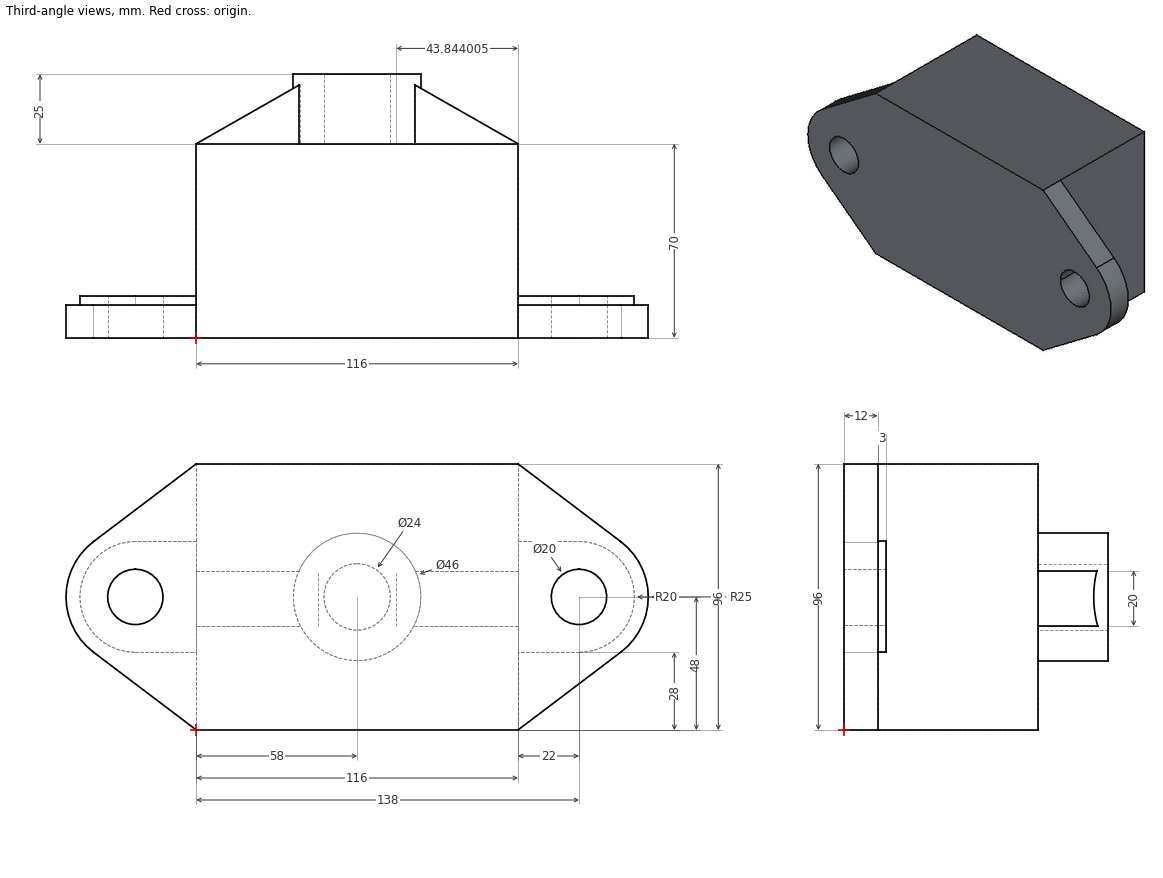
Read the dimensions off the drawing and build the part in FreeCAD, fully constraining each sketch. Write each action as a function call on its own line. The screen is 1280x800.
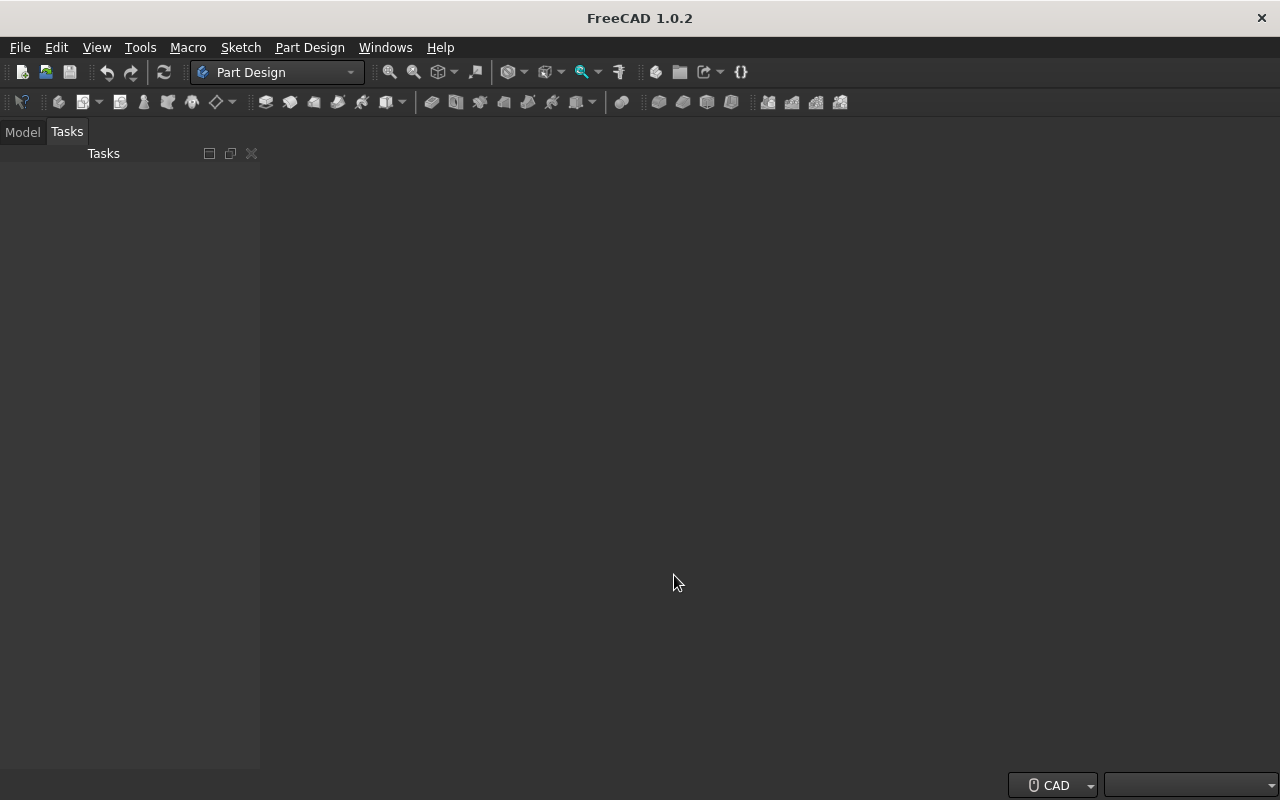
click(22, 72)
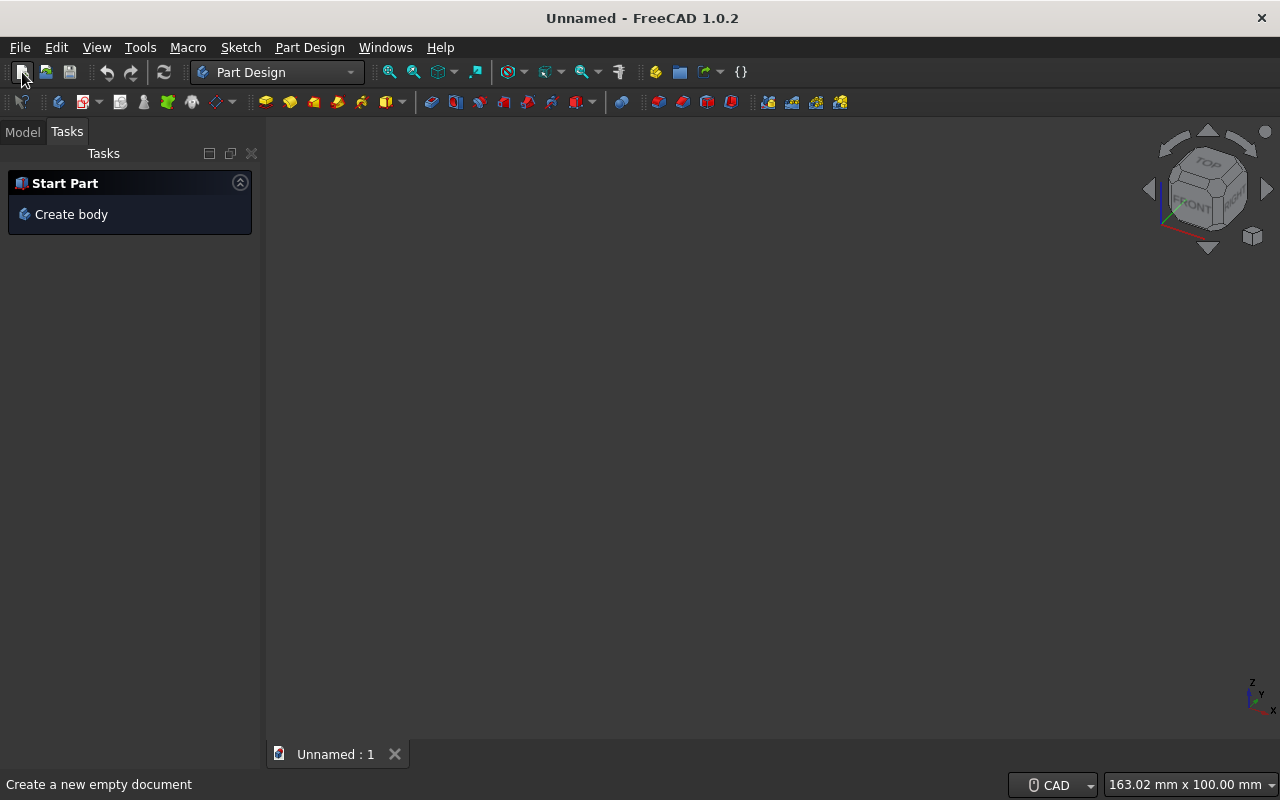
click(84, 102)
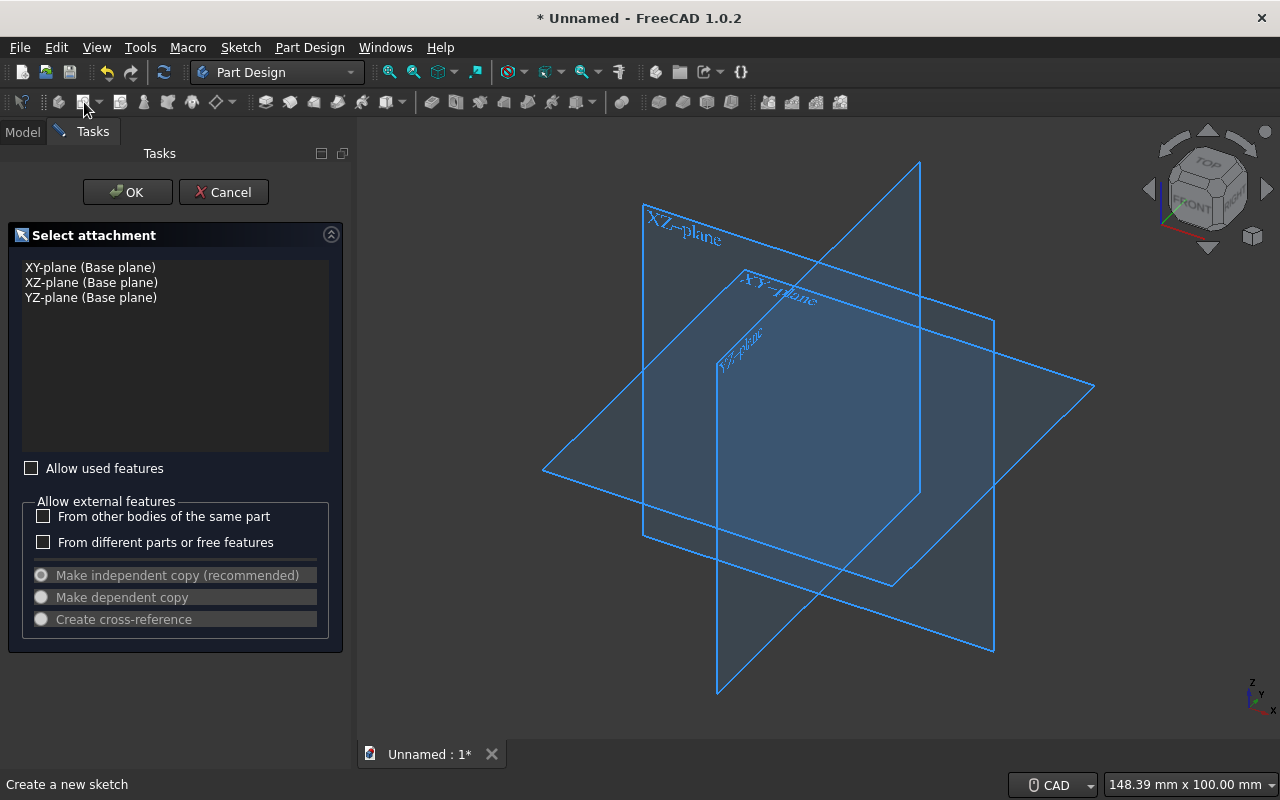
click(82, 268)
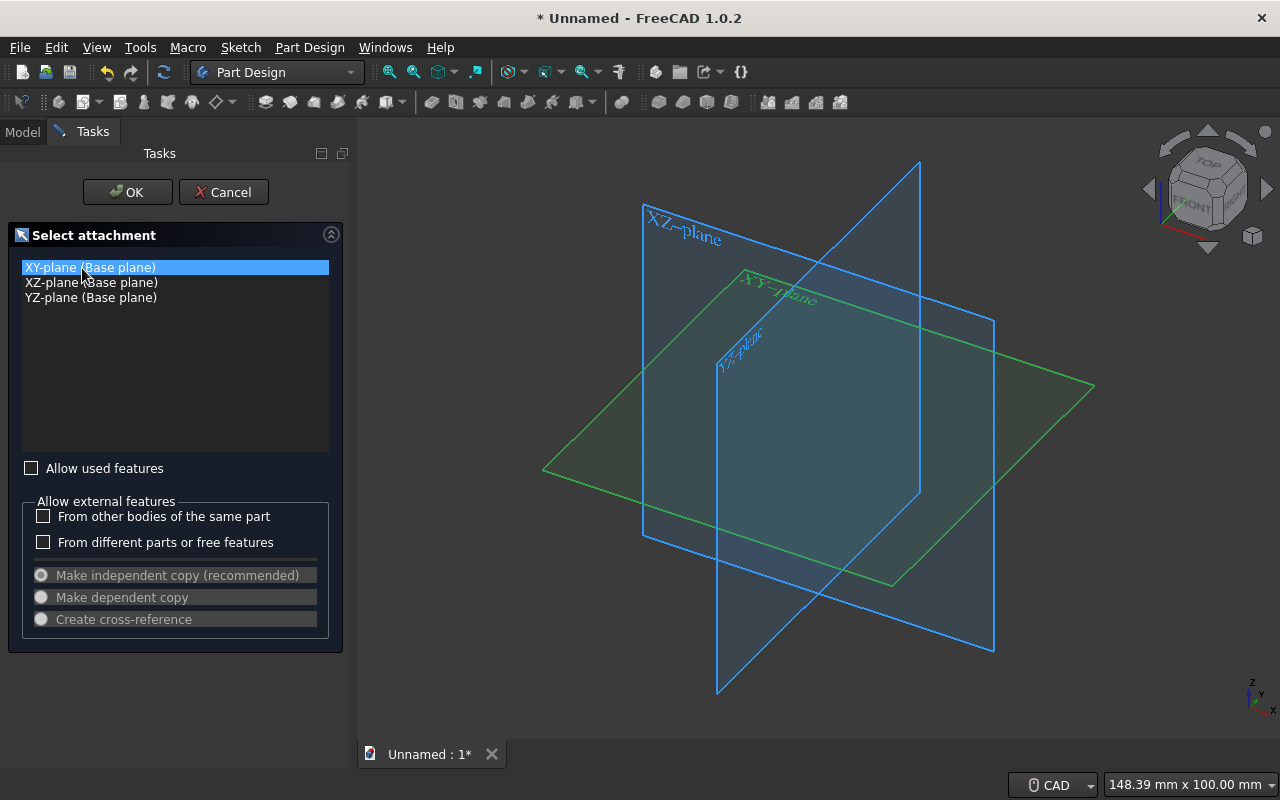
click(128, 192)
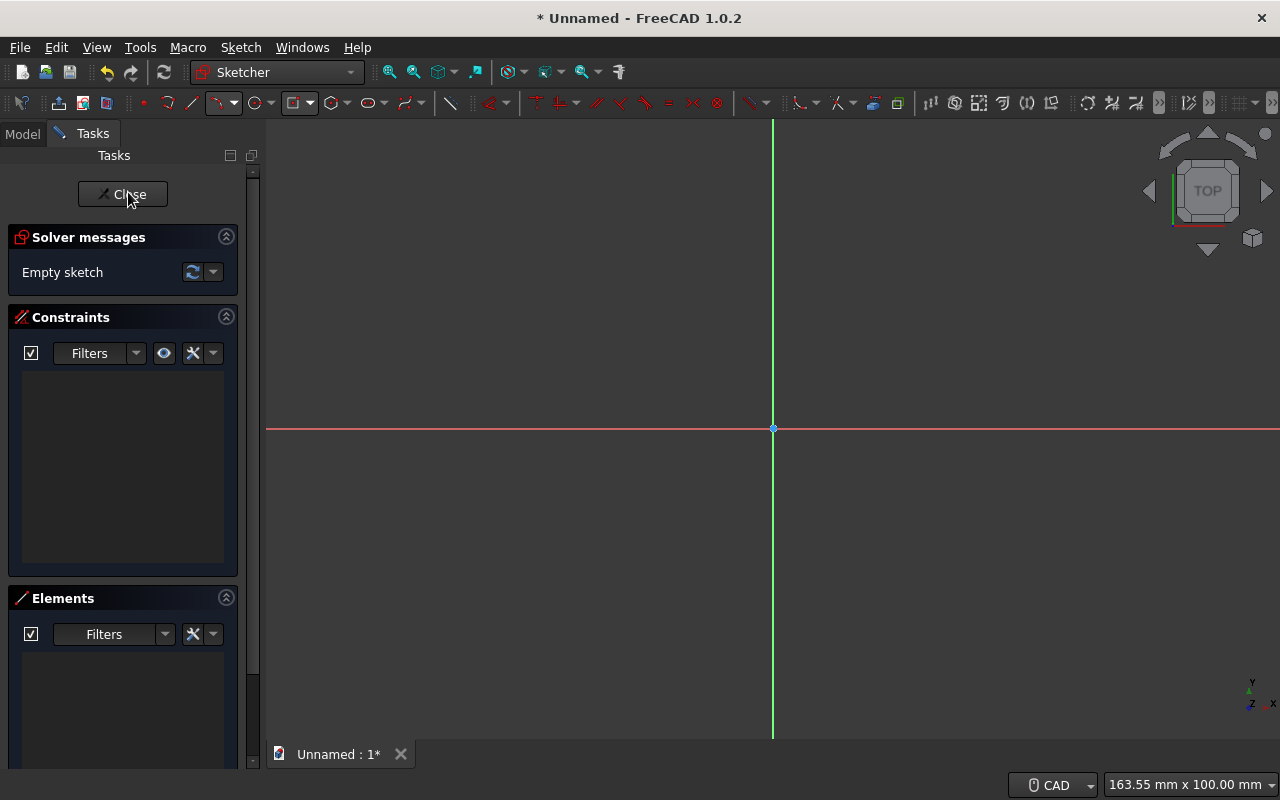
scroll(294, 693, down, 3)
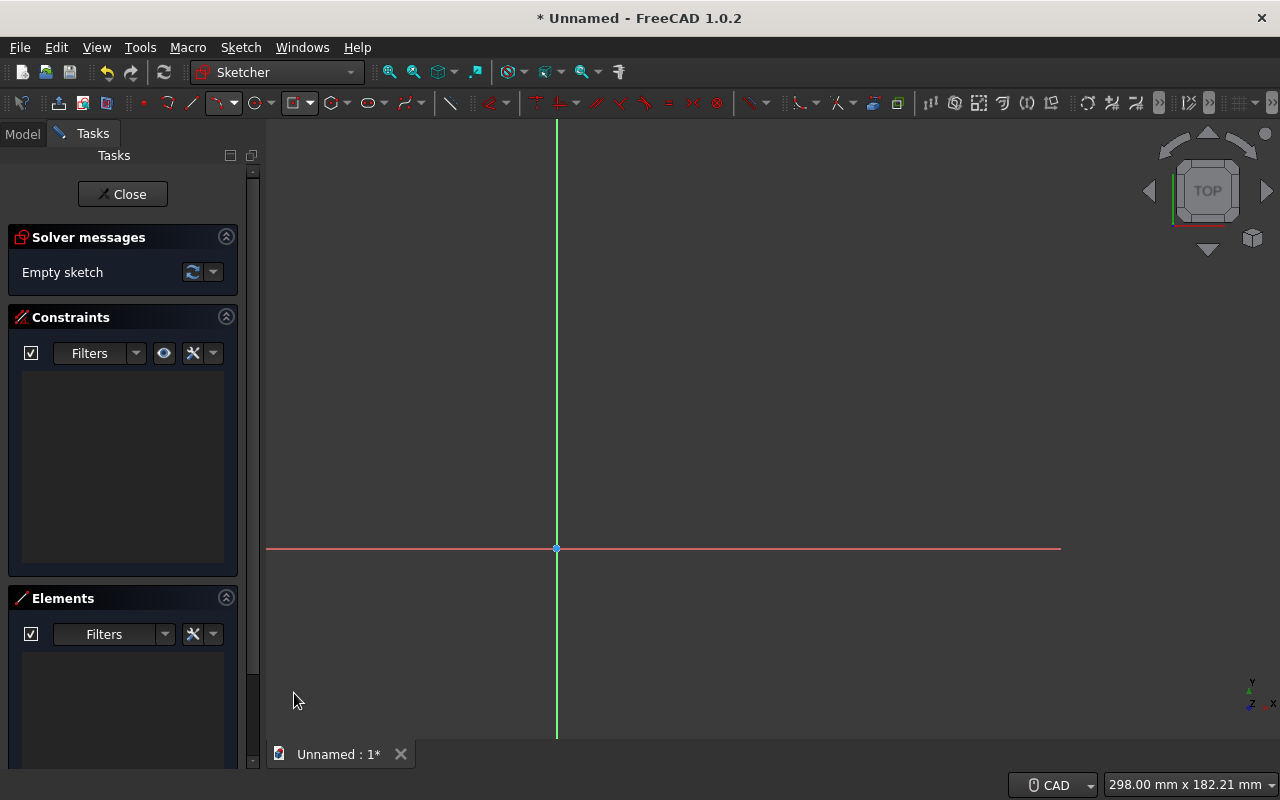
scroll(855, 430, up, 2)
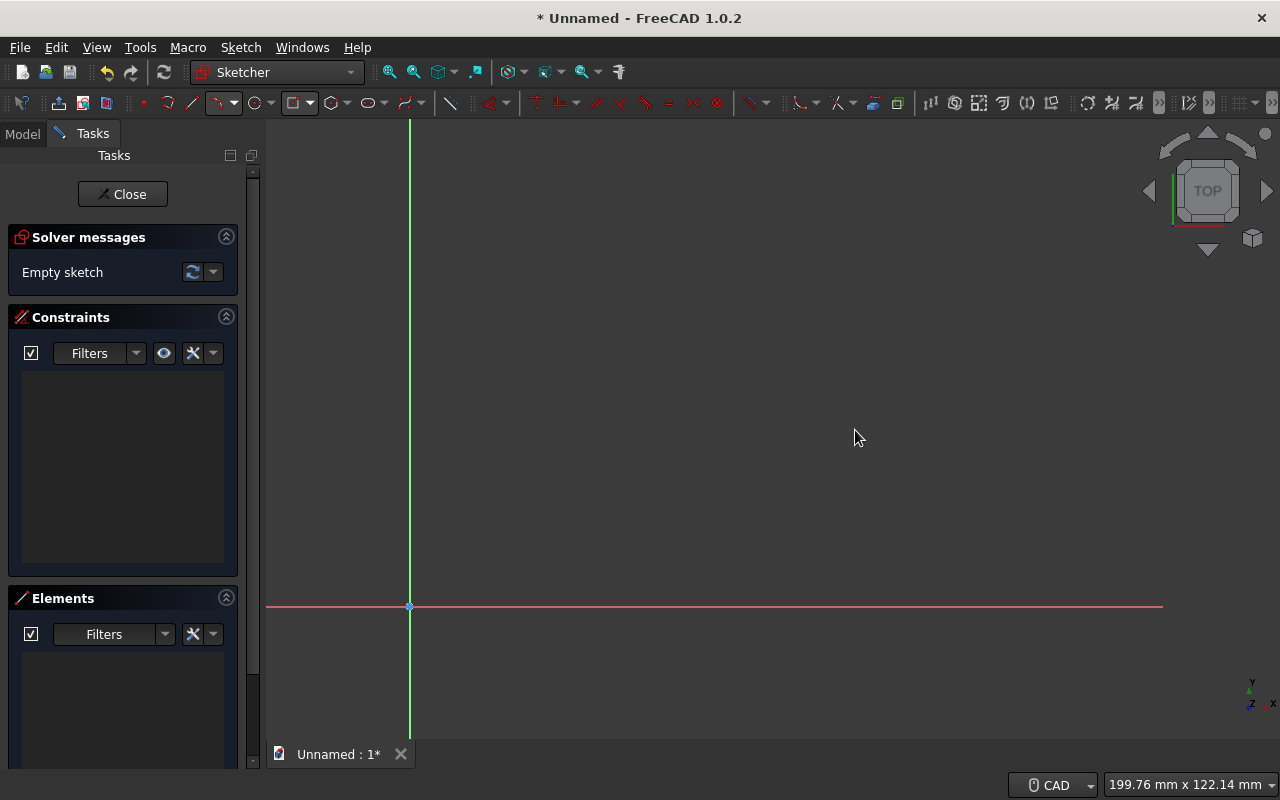
key(g)
key(r)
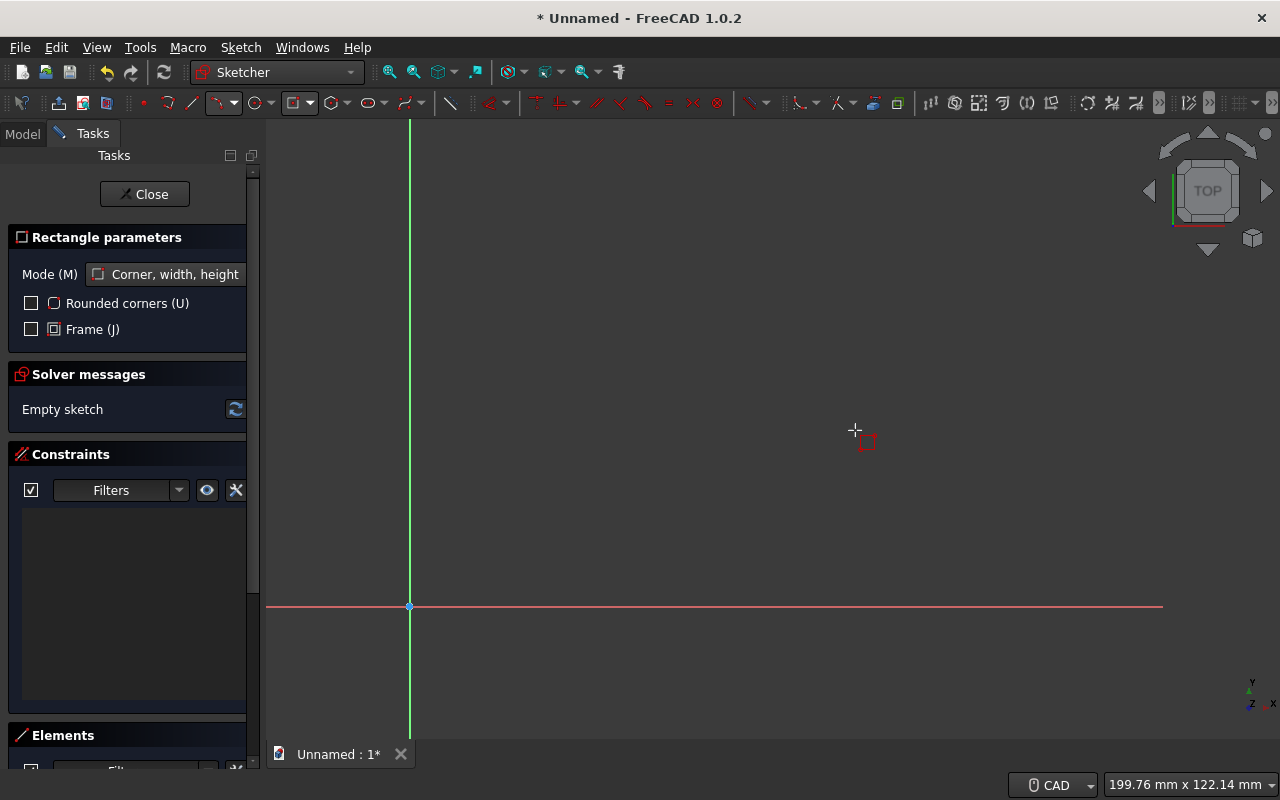
click(410, 607)
move(999, 251)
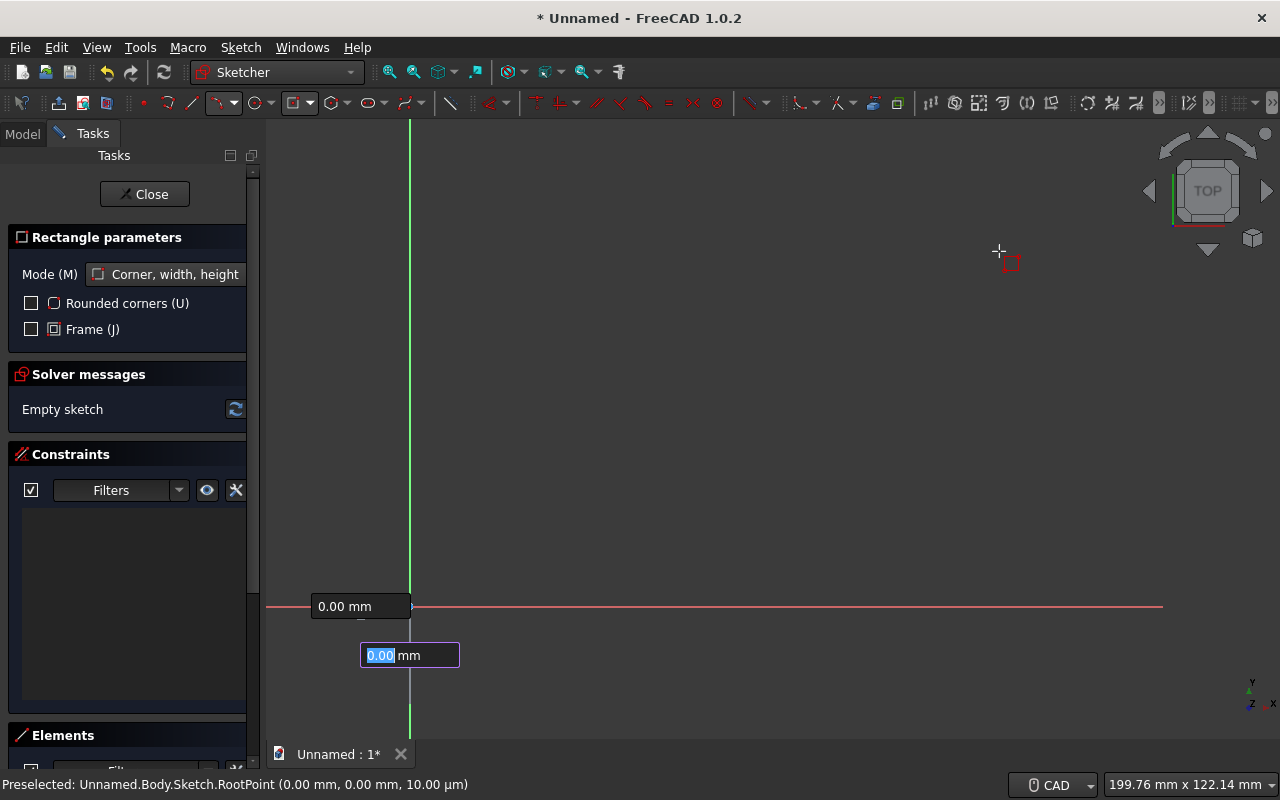
text(116)
key(Tab)
text(70)
key(Return)
key(Escape)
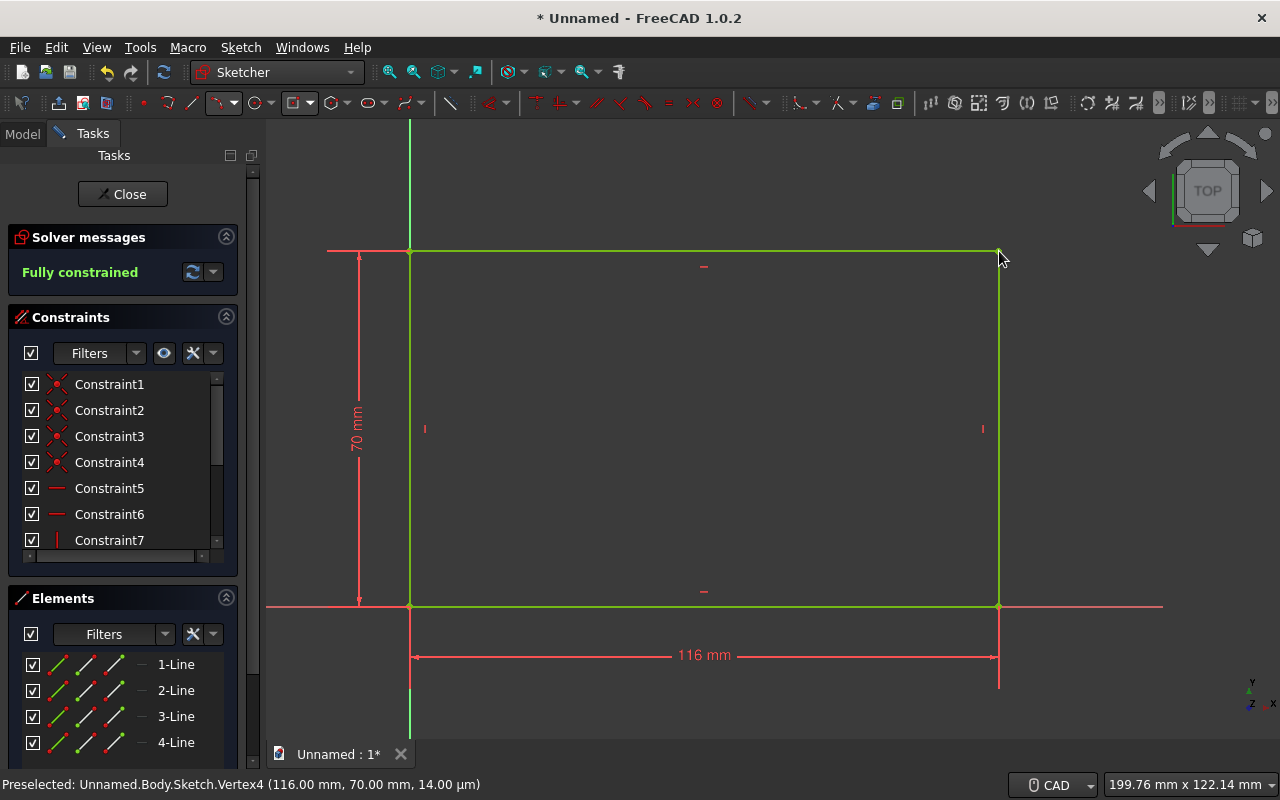
click(123, 194)